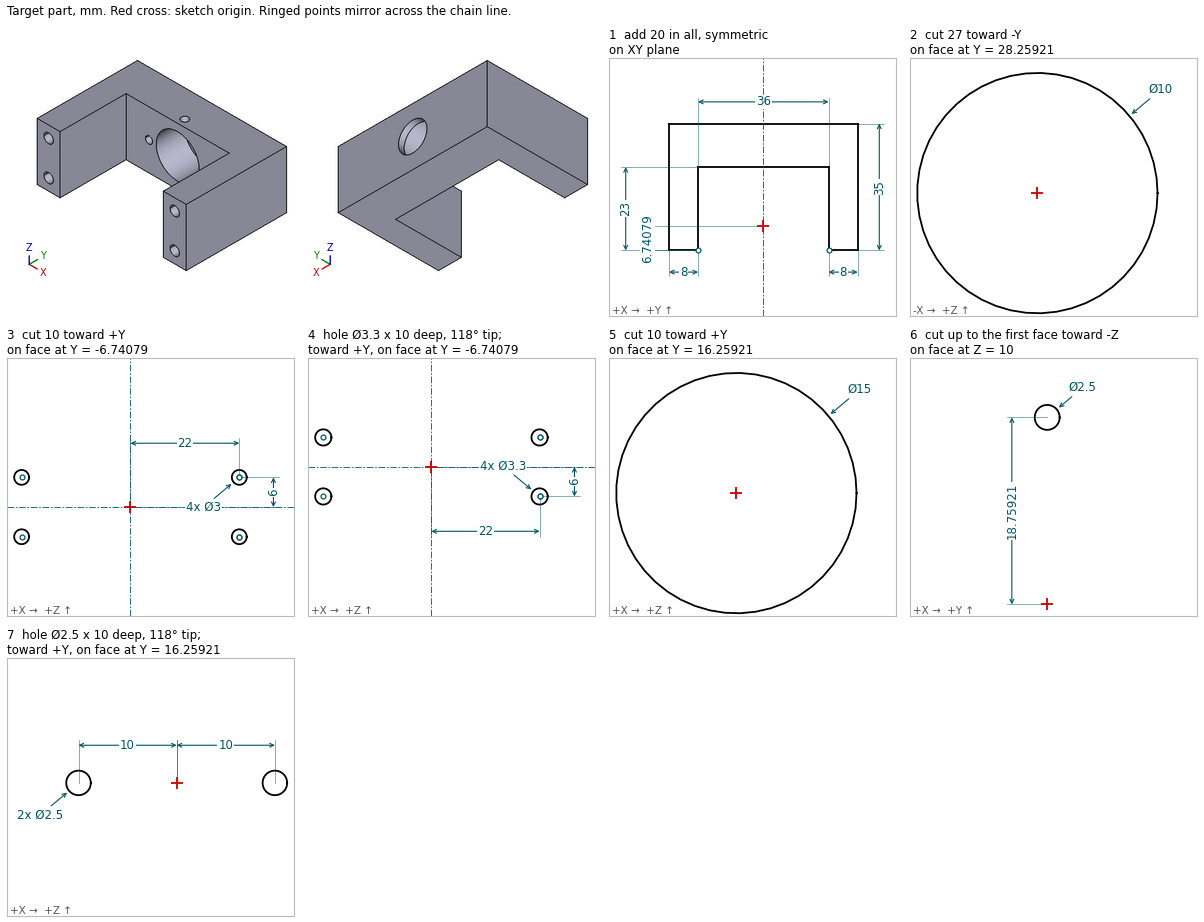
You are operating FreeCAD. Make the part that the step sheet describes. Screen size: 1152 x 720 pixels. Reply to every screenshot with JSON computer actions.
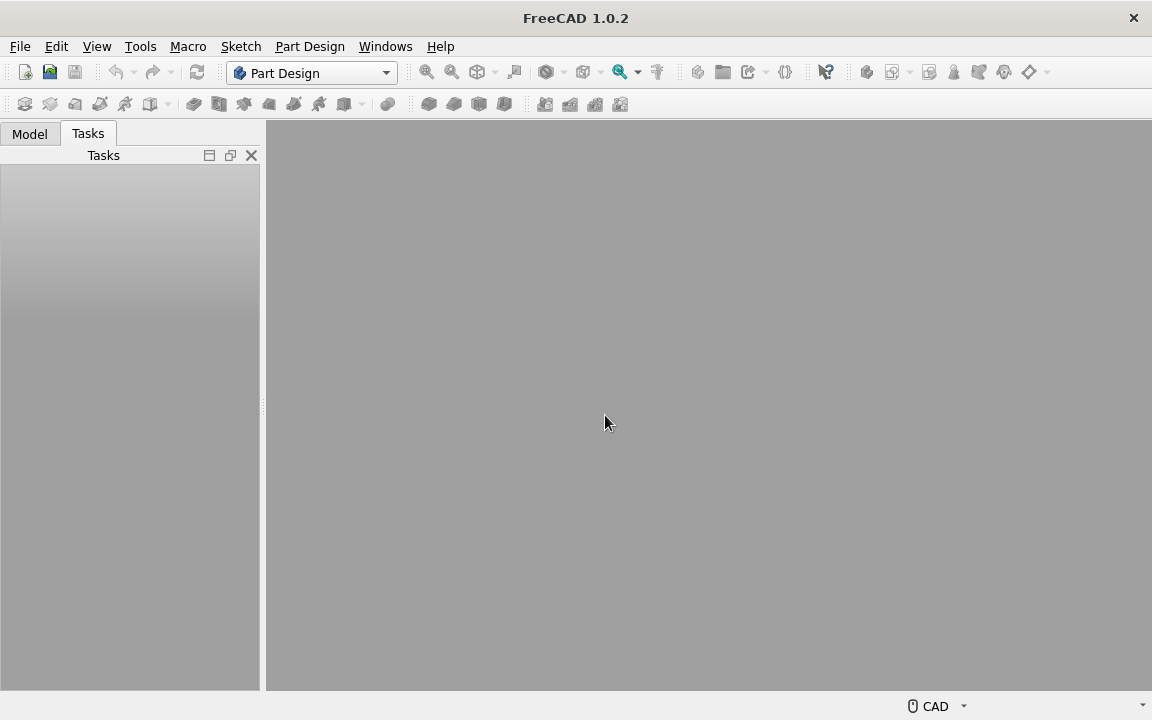
{"action": "key", "text": "ctrl+n"}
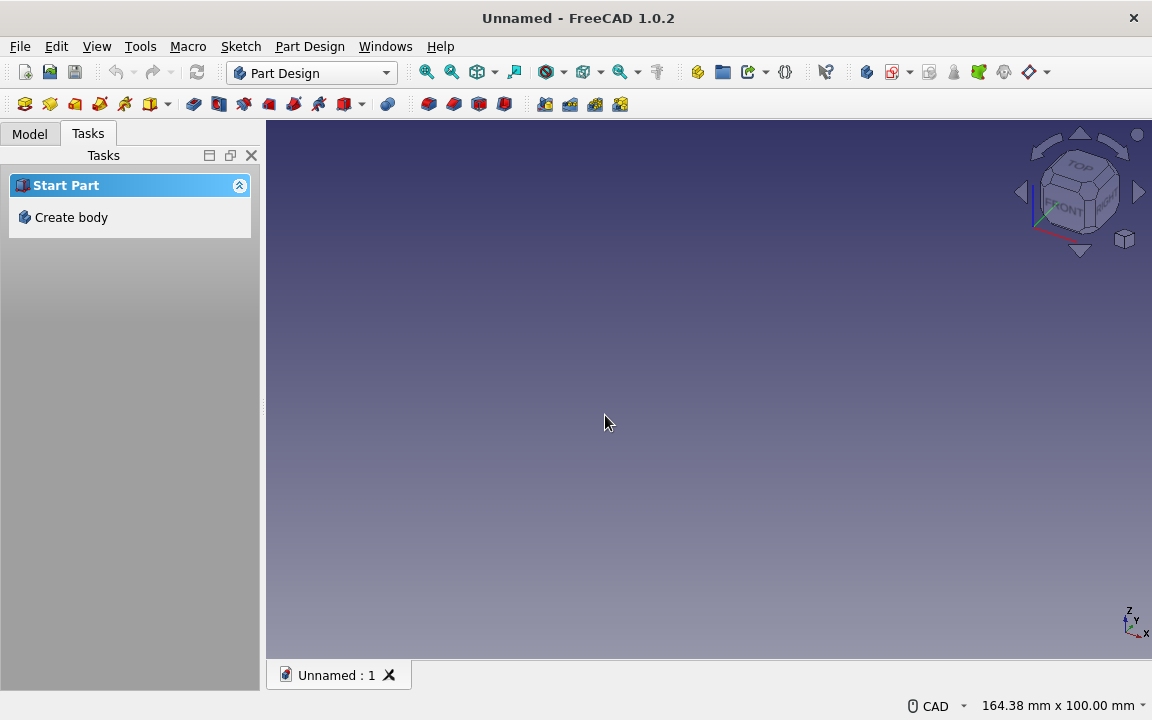
{"action": "left_click", "coordinate": [892, 72]}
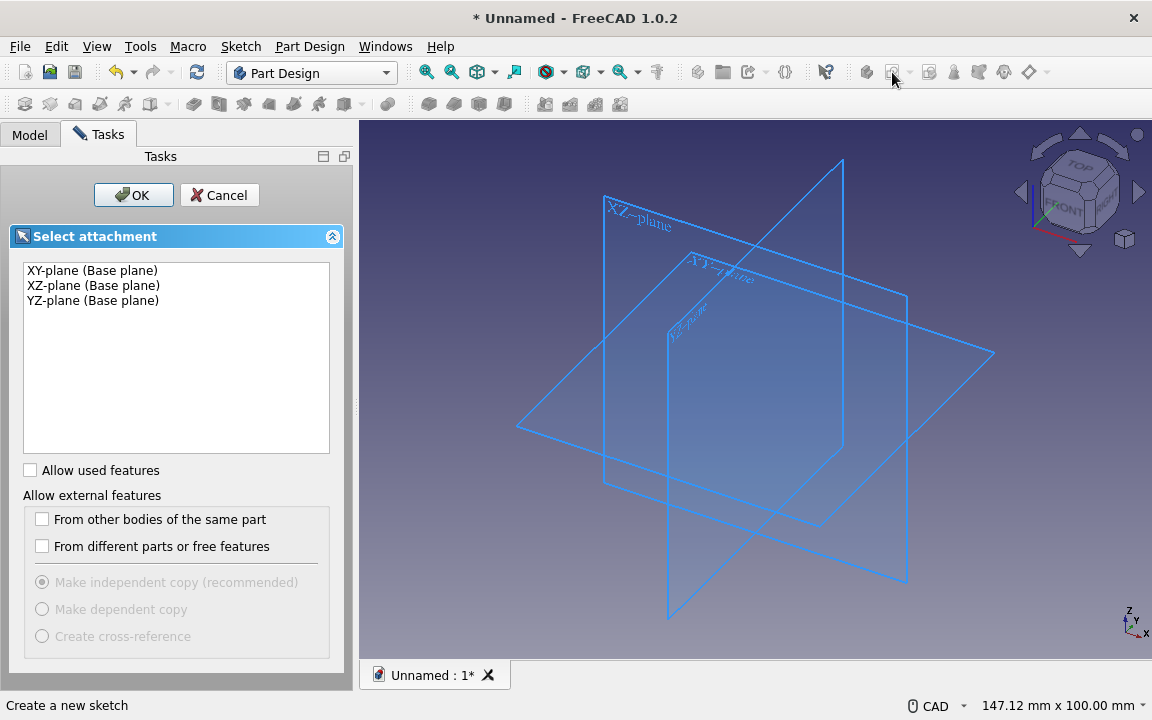
{"action": "left_click", "coordinate": [84, 270]}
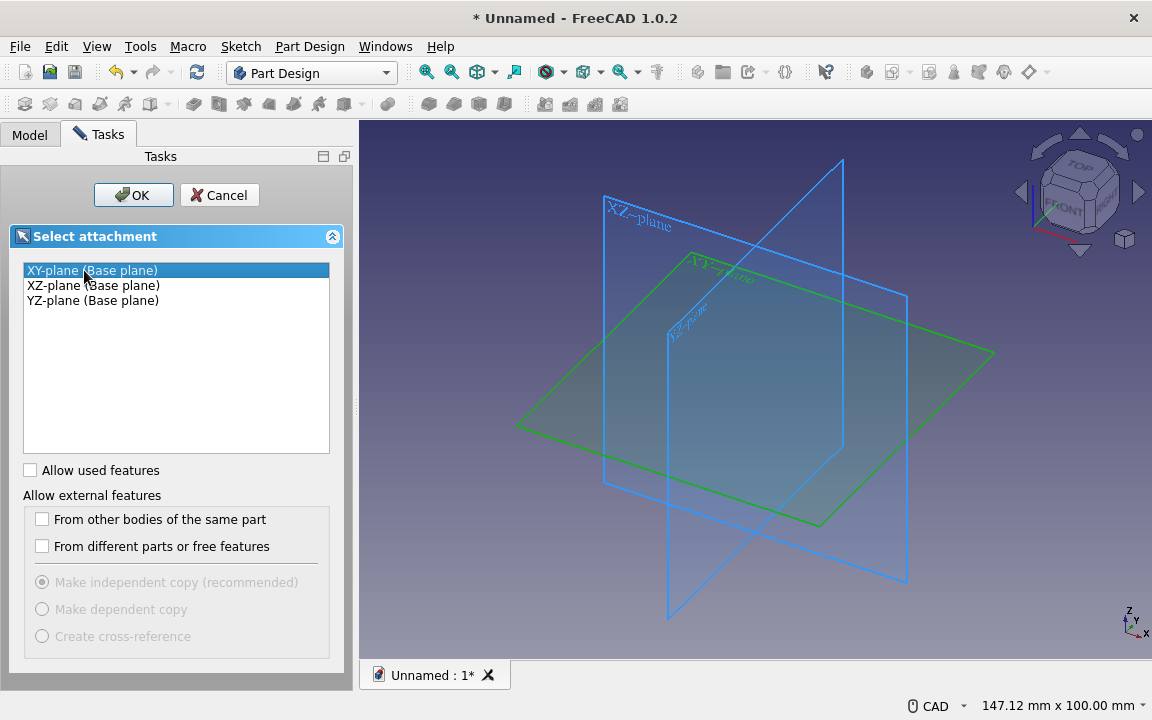
{"action": "left_click", "coordinate": [134, 195]}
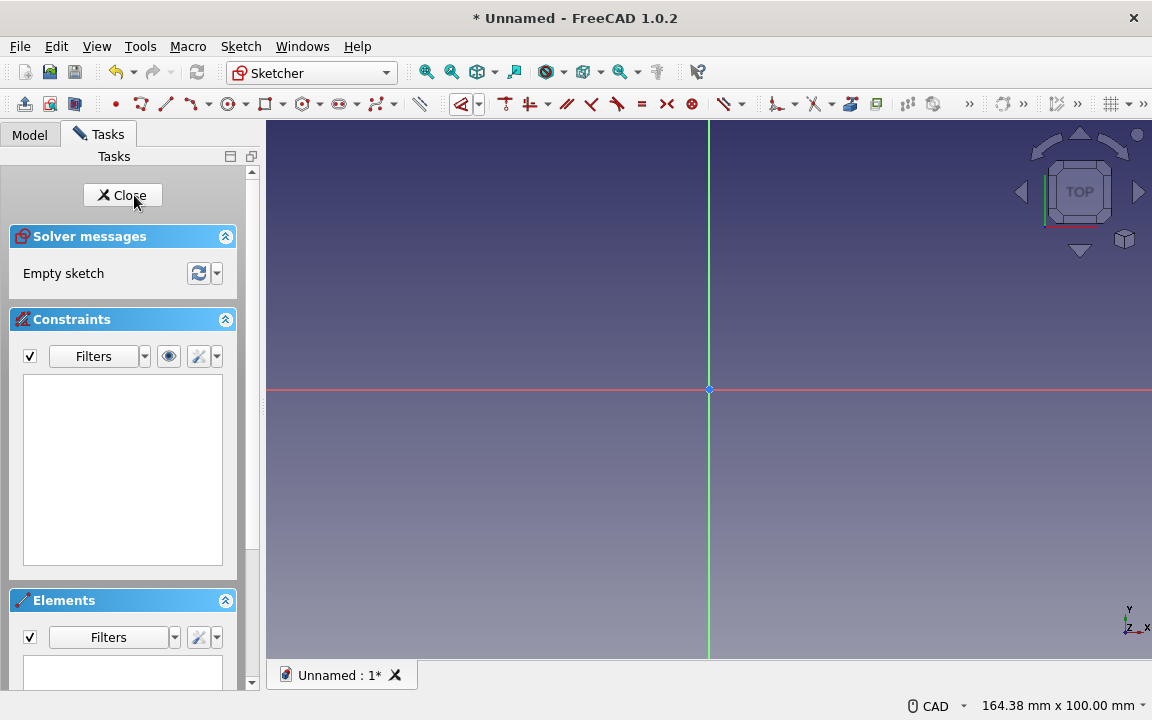
{"action": "scroll", "coordinate": [792, 261], "scroll_direction": "up", "scroll_amount": 3}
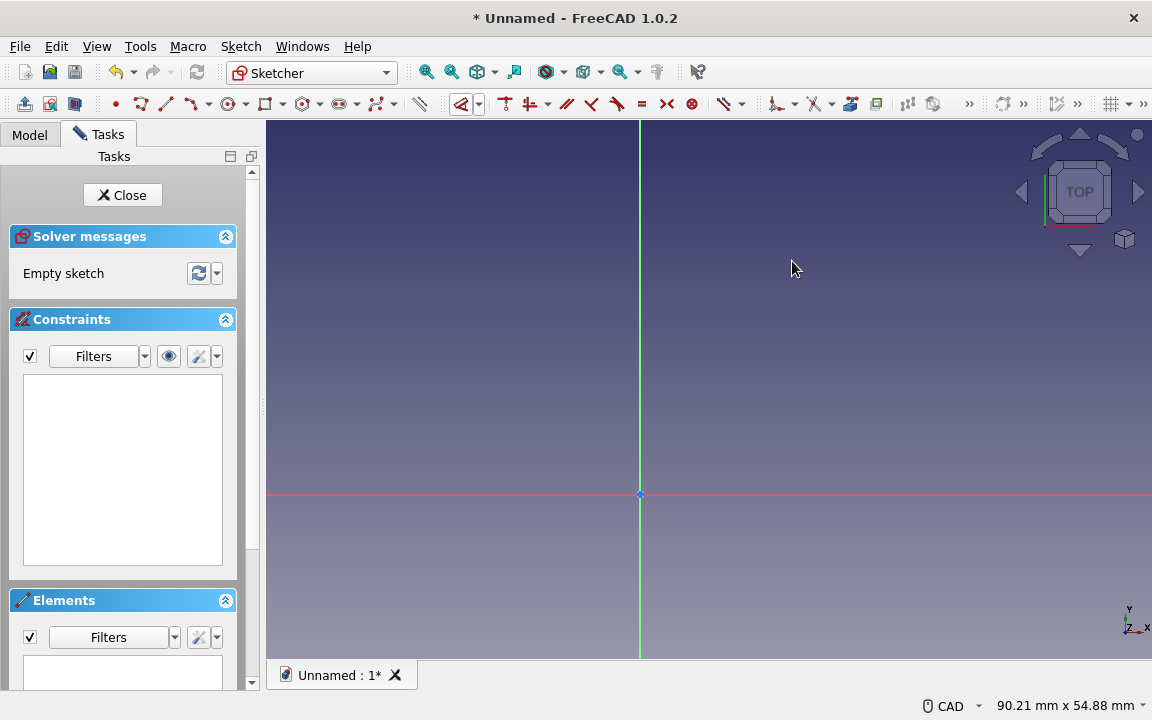
{"action": "left_click", "coordinate": [141, 104]}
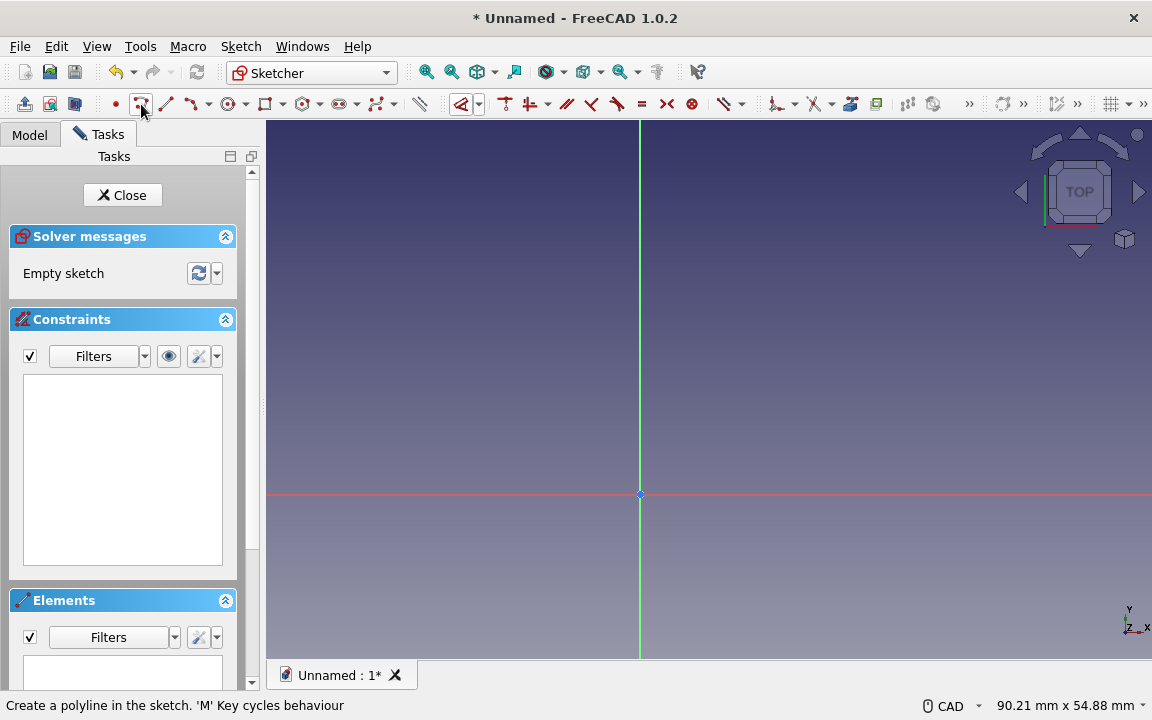
{"action": "left_click", "coordinate": [463, 561]}
{"action": "left_click", "coordinate": [463, 335]}
{"action": "left_click", "coordinate": [817, 335]}
{"action": "left_click", "coordinate": [817, 561]}
{"action": "left_click", "coordinate": [896, 561]}
{"action": "left_click", "coordinate": [896, 217]}
{"action": "left_click", "coordinate": [385, 217]}
{"action": "left_click", "coordinate": [385, 561]}
{"action": "left_click", "coordinate": [463, 562]}
{"action": "key", "text": "Escape"}
{"action": "key", "text": "Escape"}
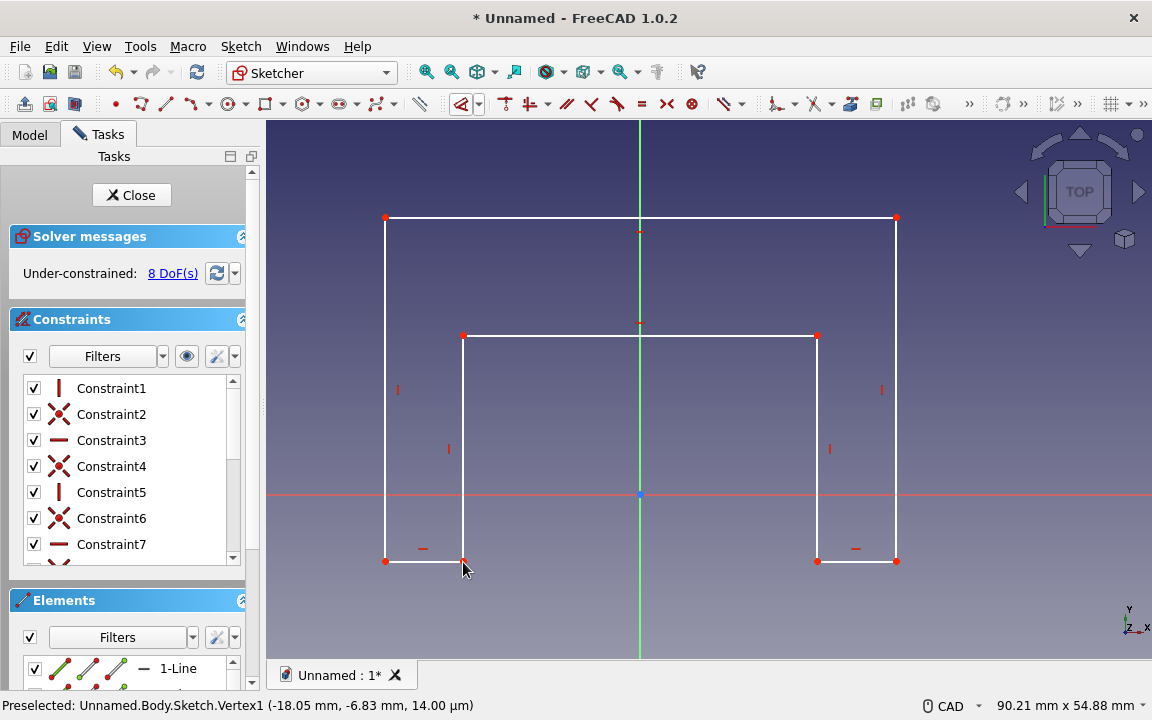
{"action": "left_click", "coordinate": [463, 562]}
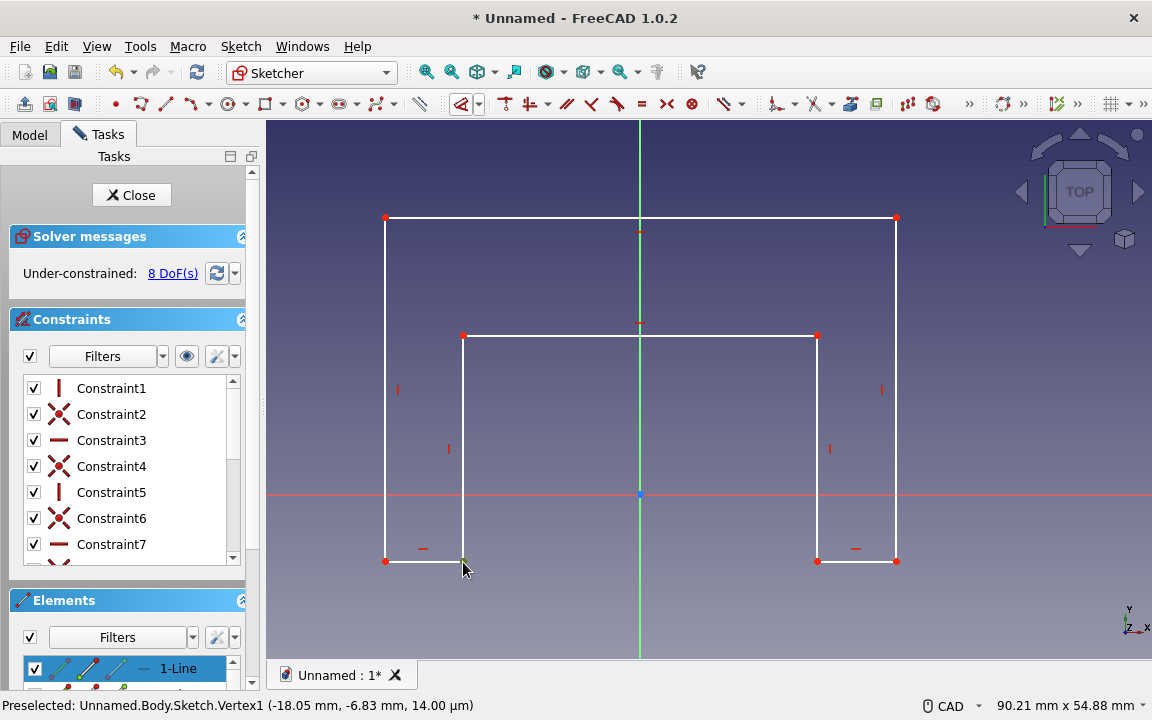
{"action": "left_click", "coordinate": [817, 562]}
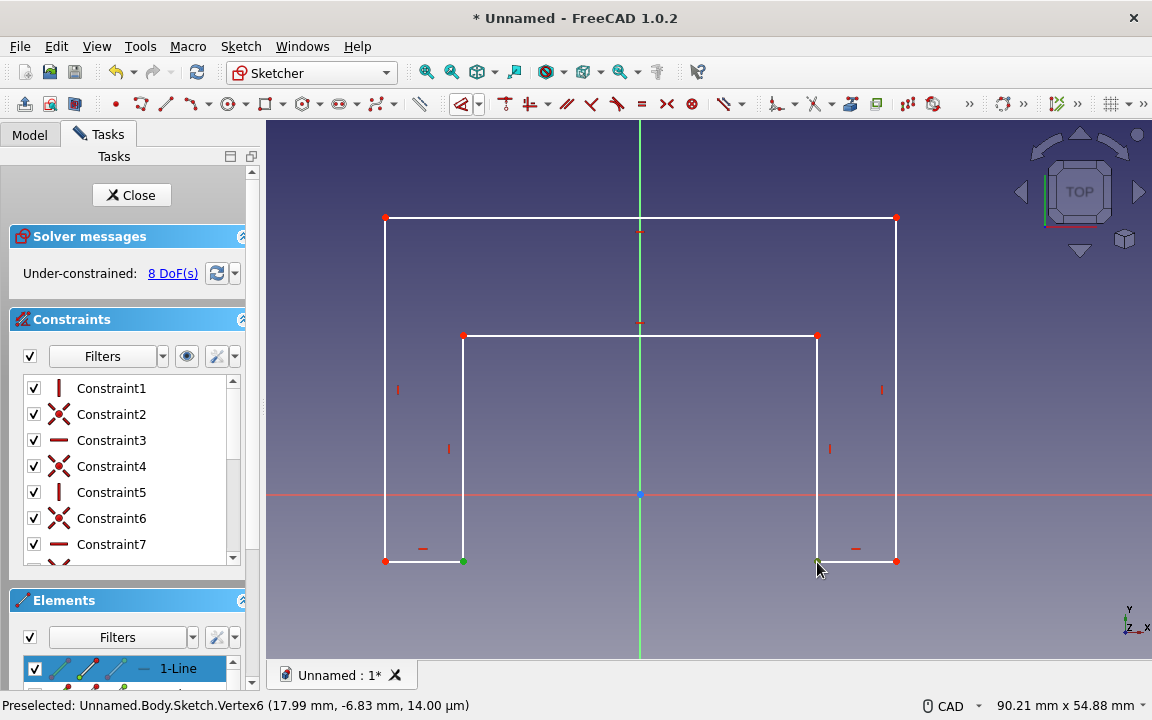
{"action": "left_click", "coordinate": [640, 596]}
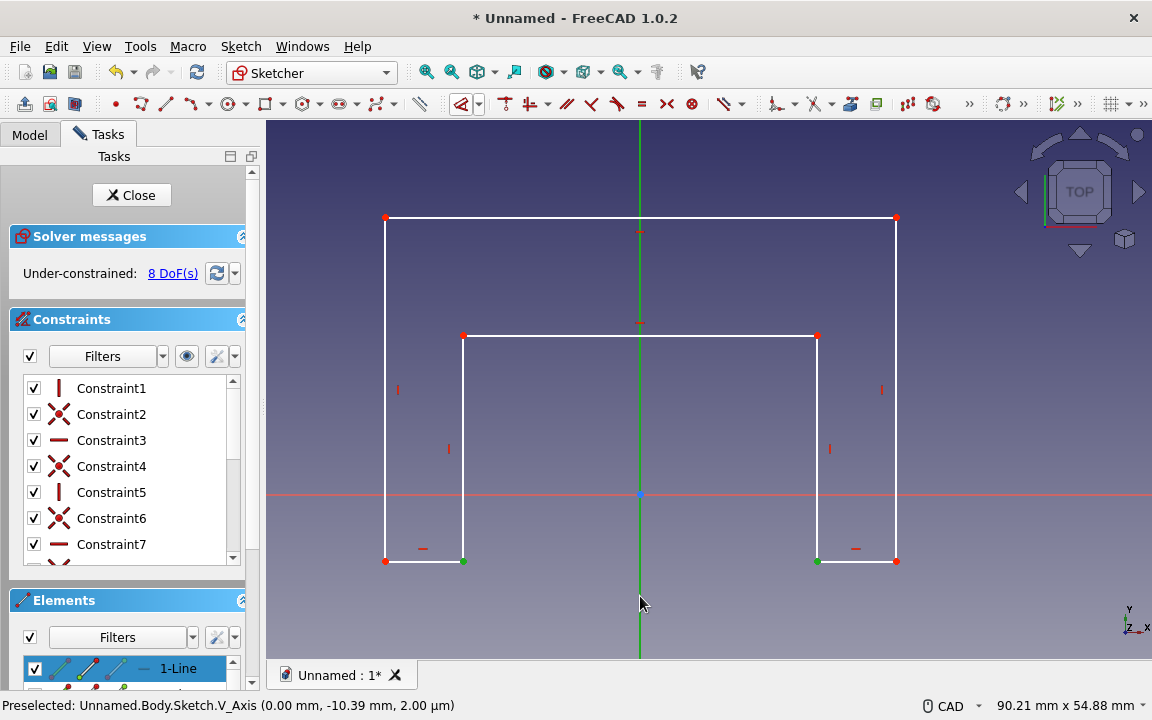
{"action": "key", "text": "s"}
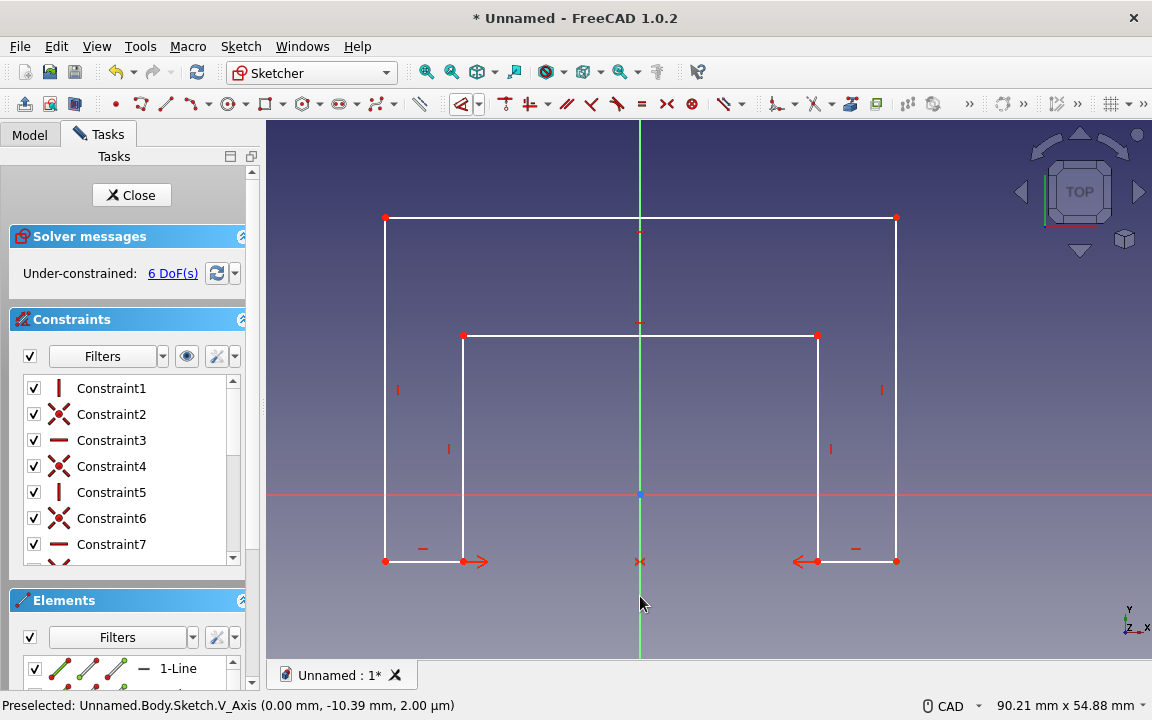
{"action": "left_click", "coordinate": [841, 562]}